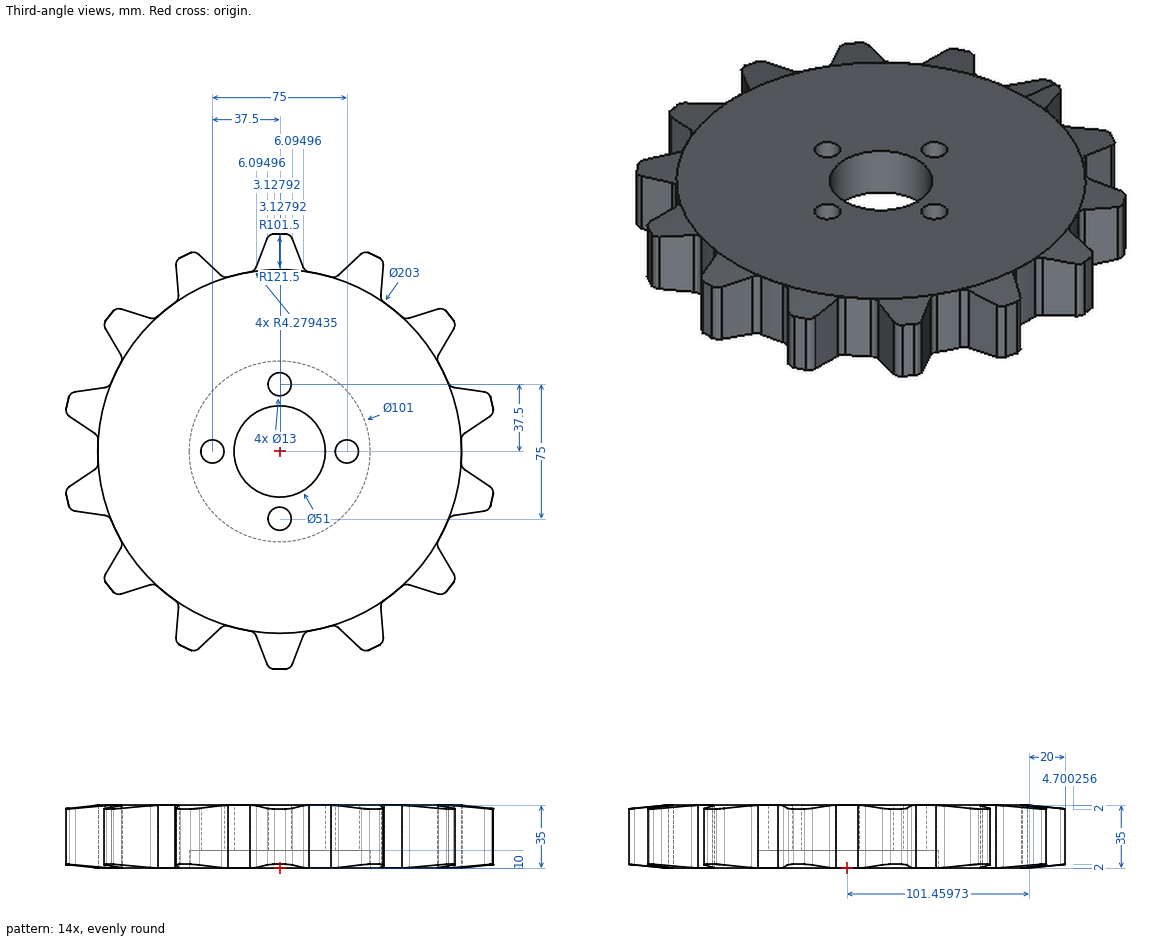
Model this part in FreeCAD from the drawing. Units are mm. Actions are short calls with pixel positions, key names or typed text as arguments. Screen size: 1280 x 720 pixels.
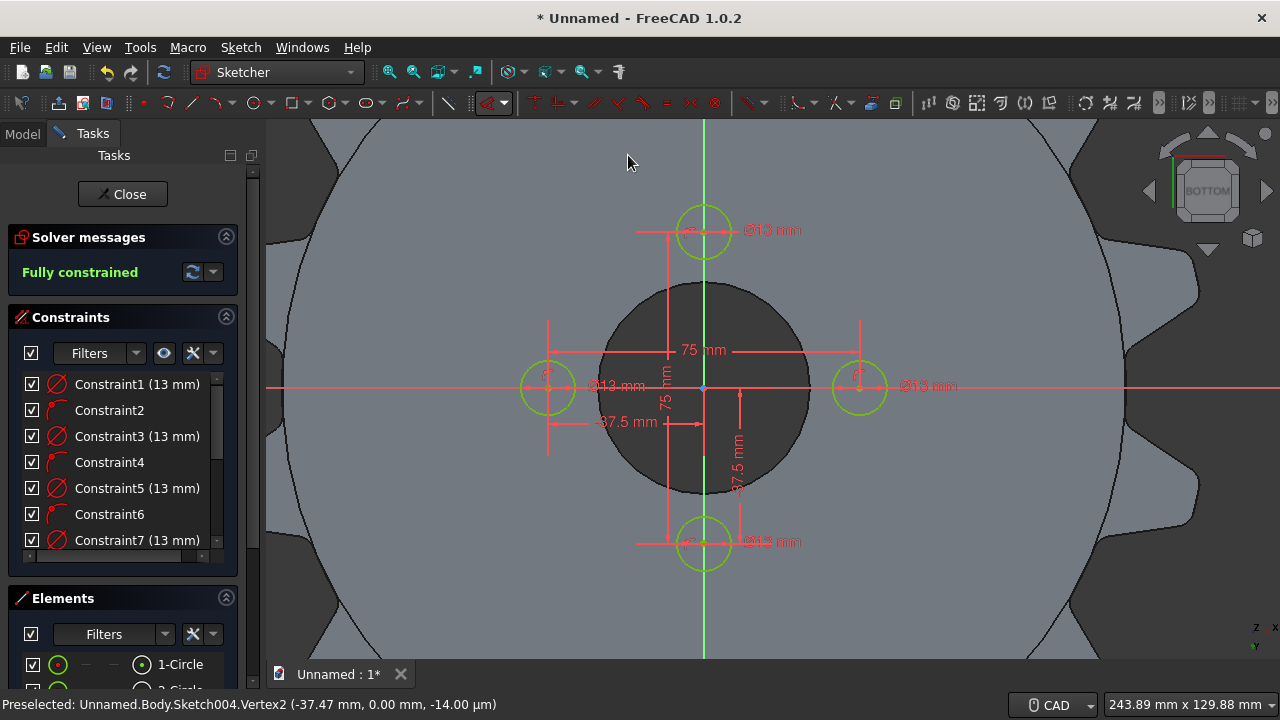
click(123, 194)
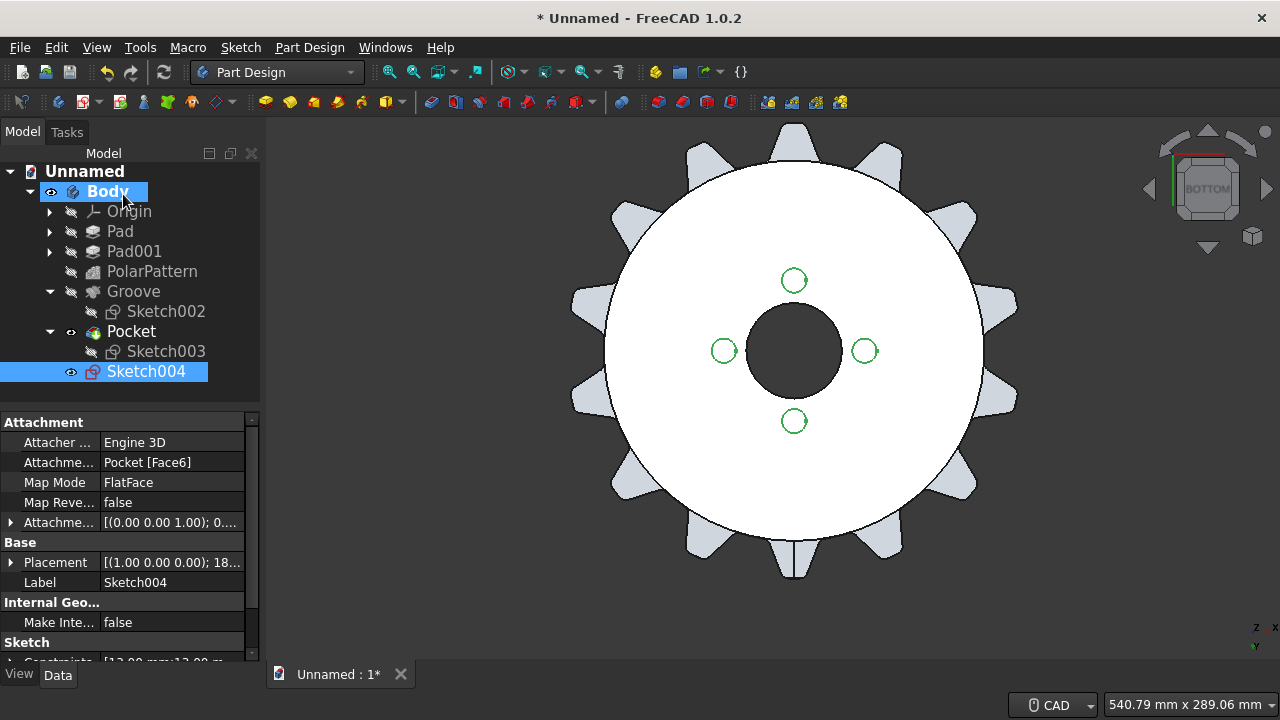
click(432, 102)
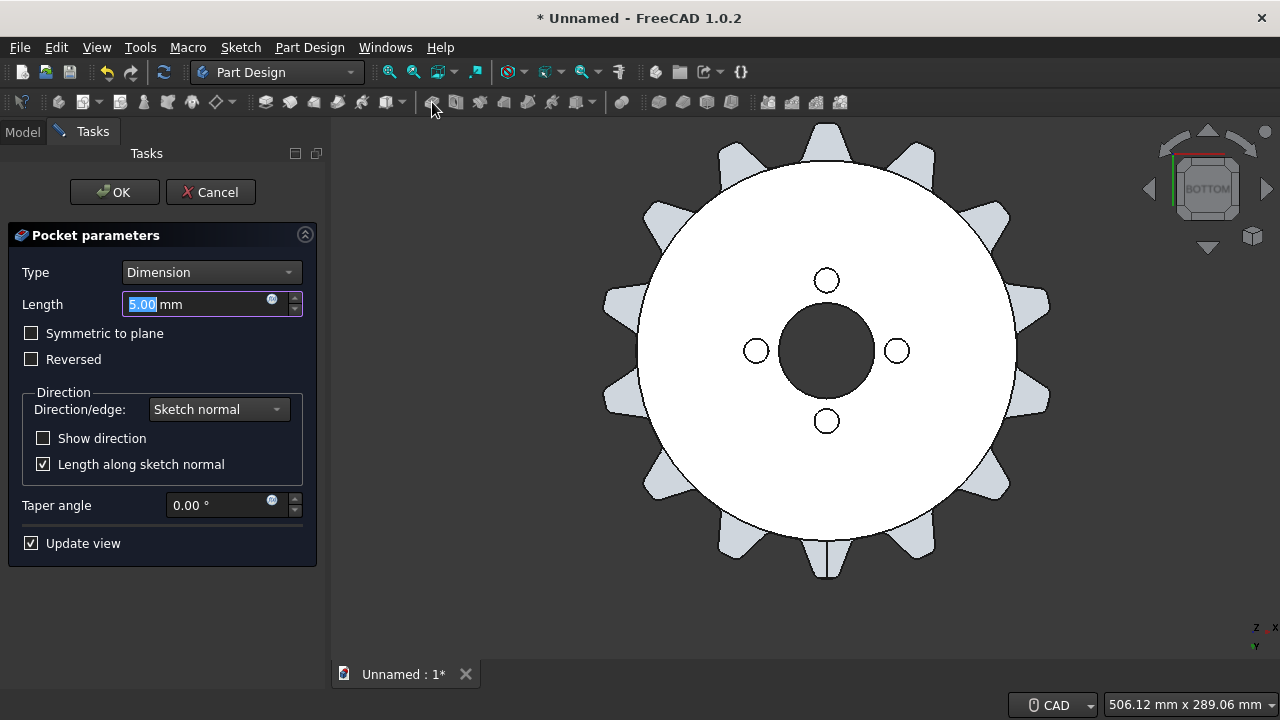
click(212, 272)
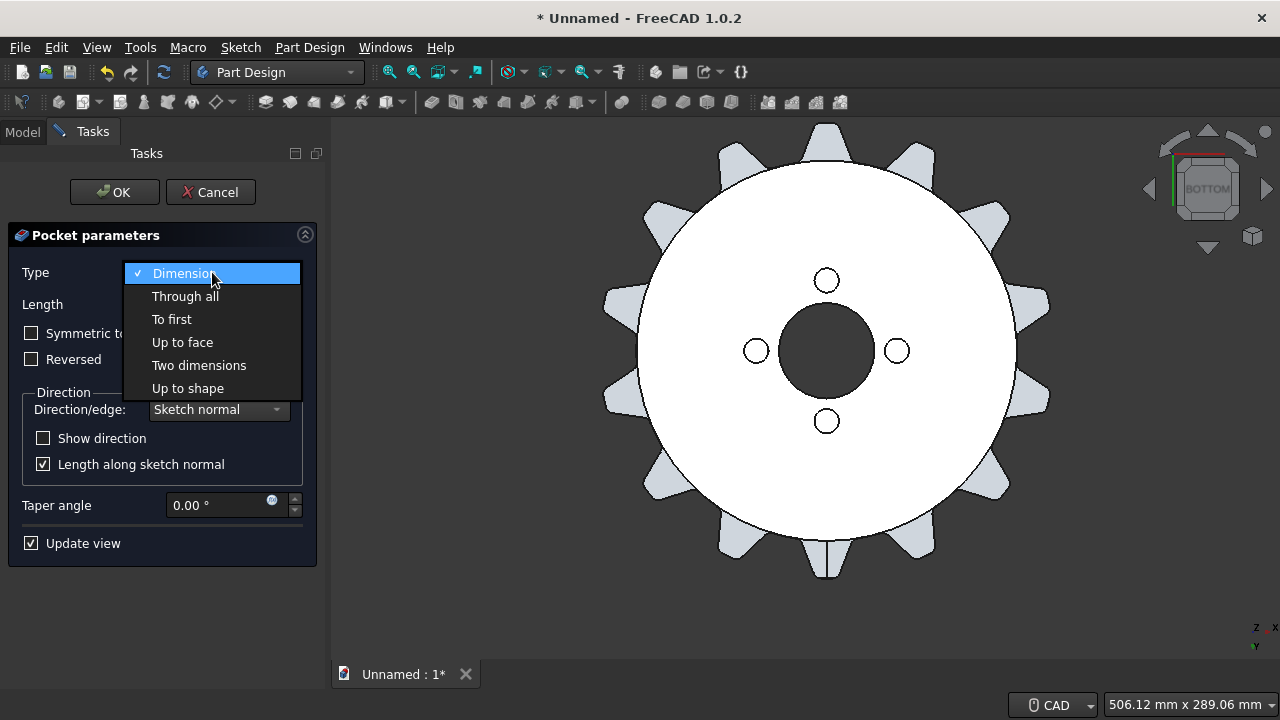
click(212, 296)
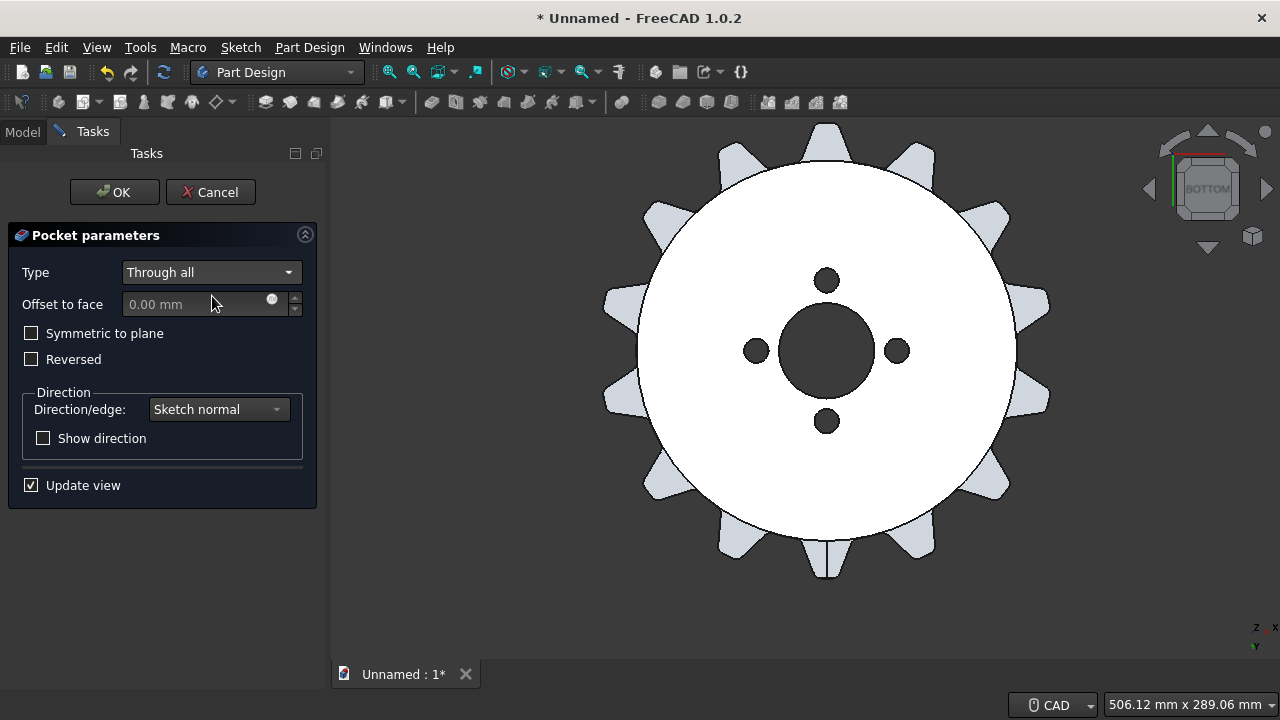
click(115, 192)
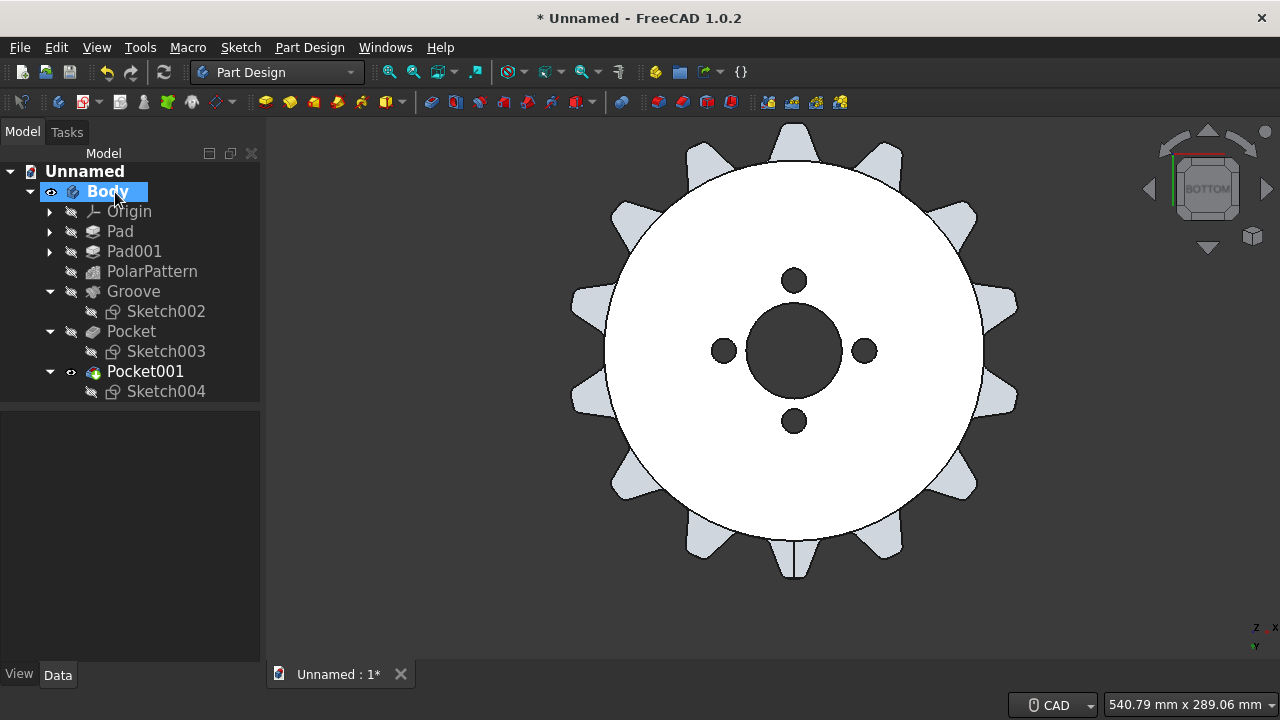
click(849, 241)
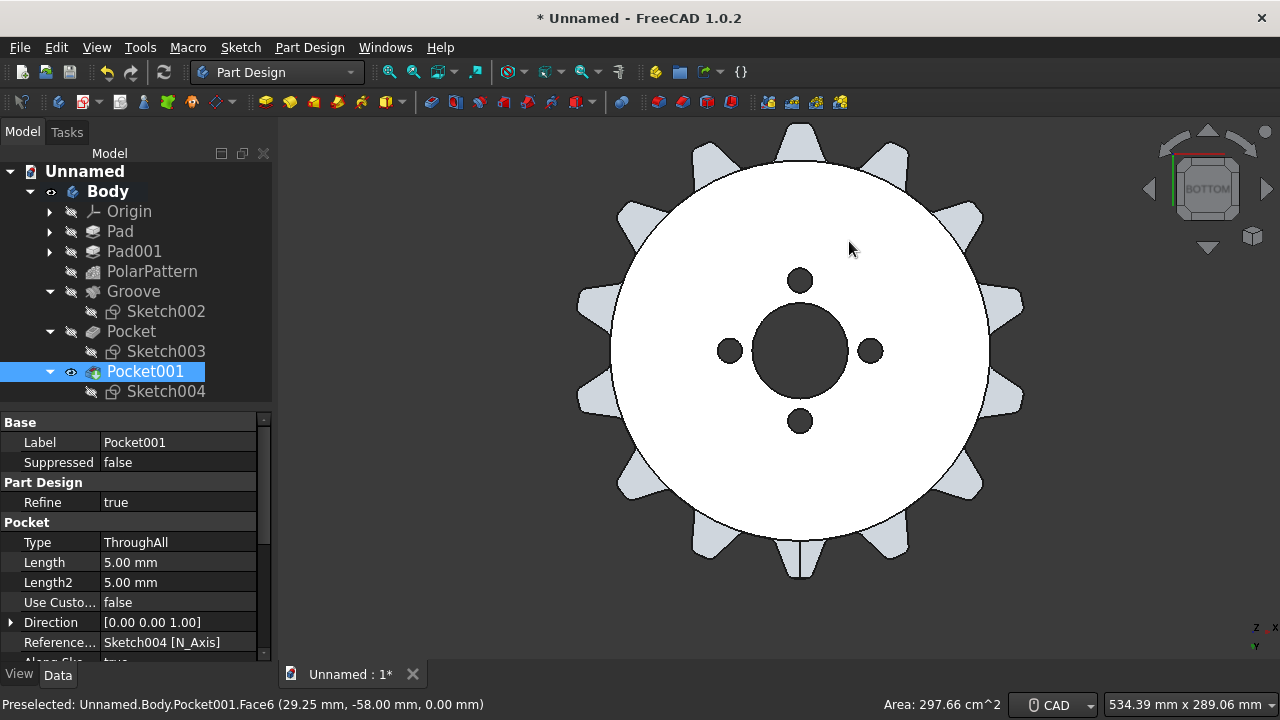
click(84, 102)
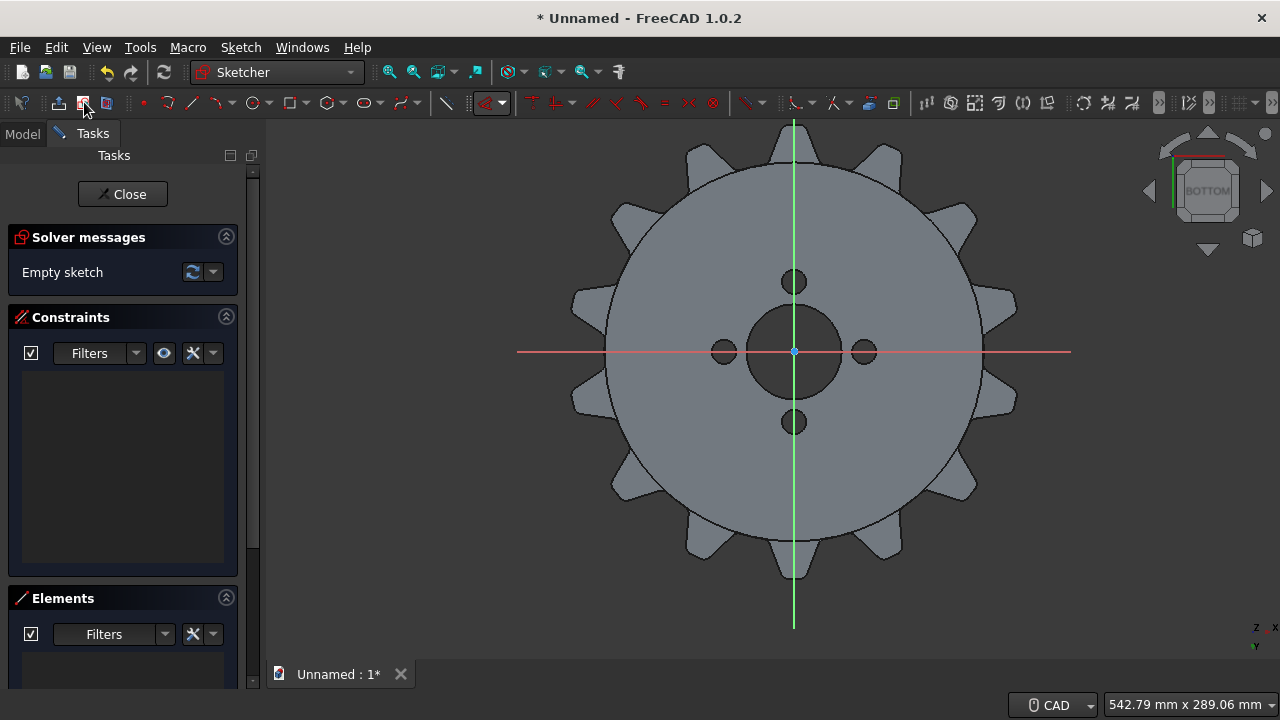
scroll(903, 307, up, 3)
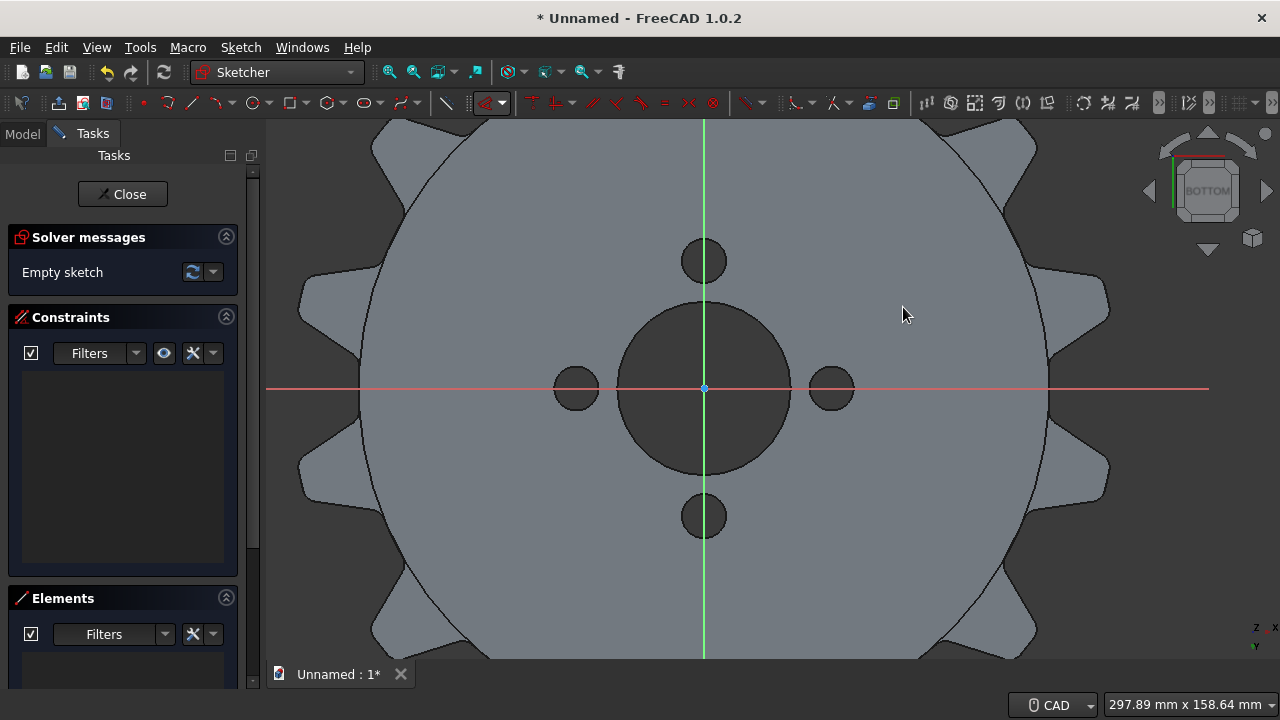
click(254, 104)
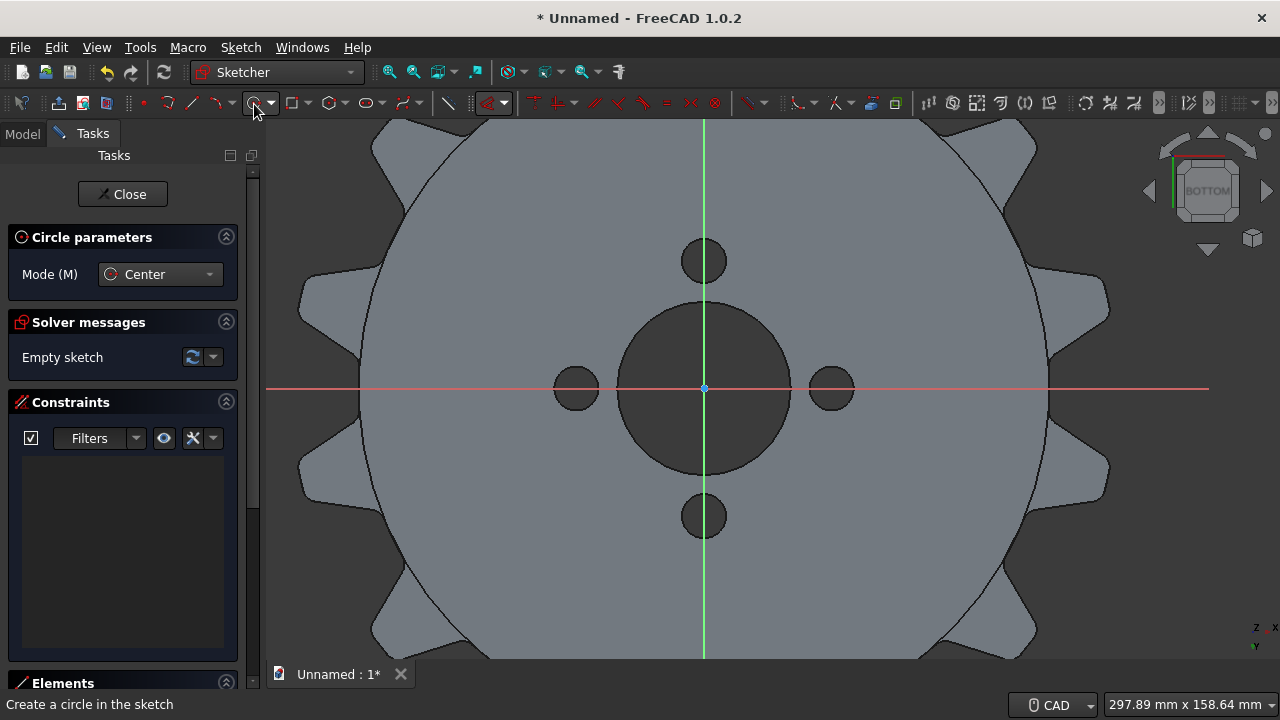
click(704, 389)
move(826, 267)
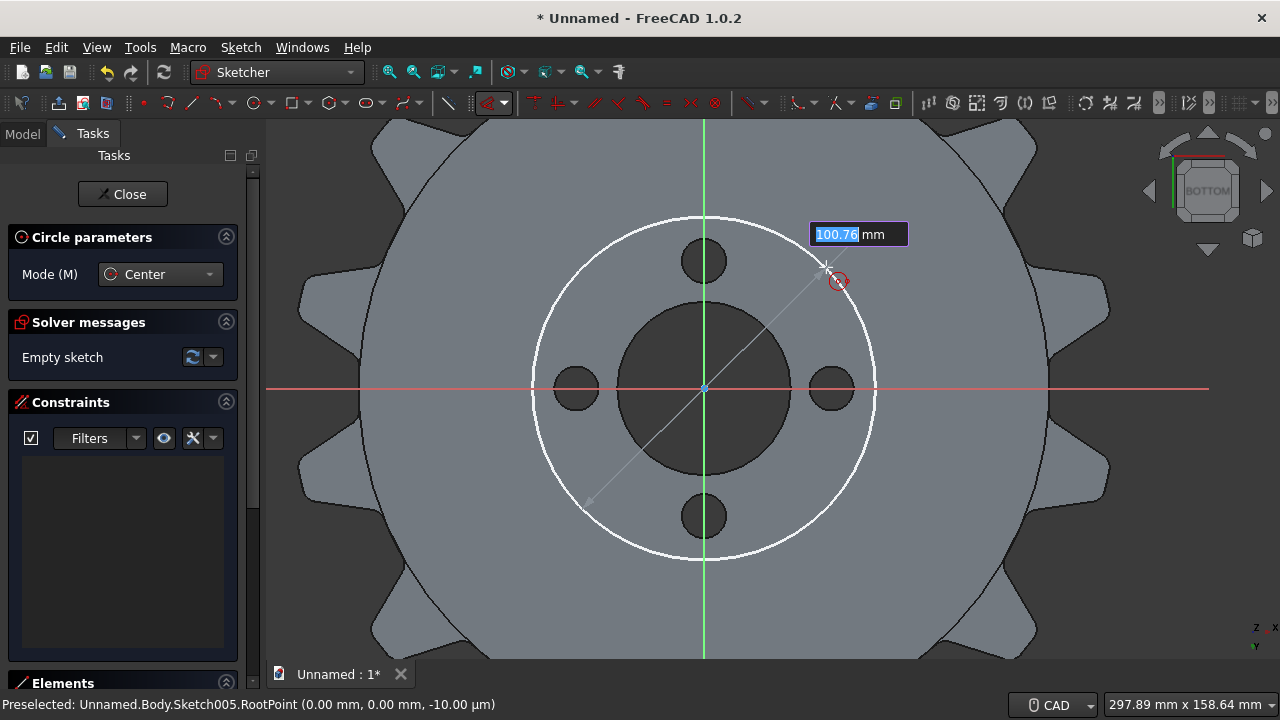
text(101)
key(Return)
key(Escape)